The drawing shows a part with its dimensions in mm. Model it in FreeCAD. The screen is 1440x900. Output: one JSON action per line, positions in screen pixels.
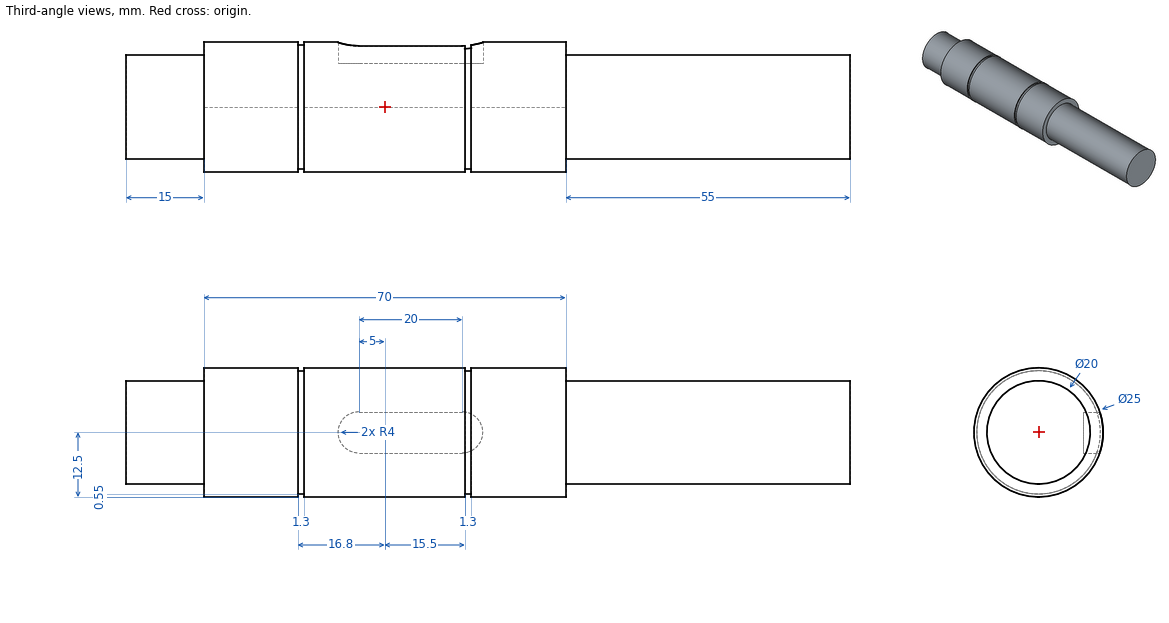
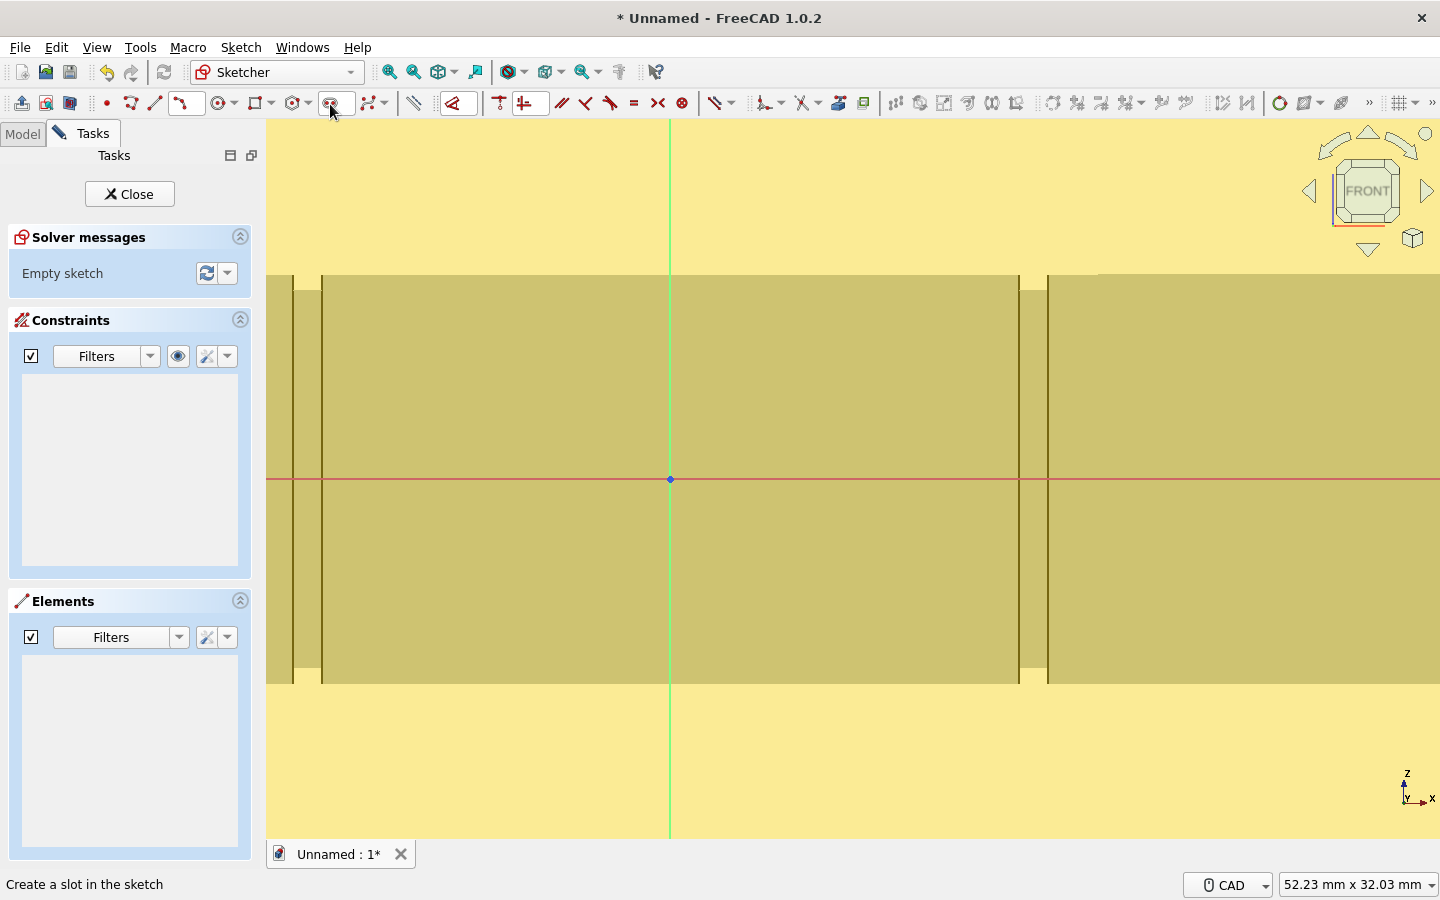
{"action": "left_click", "coordinate": [558, 479]}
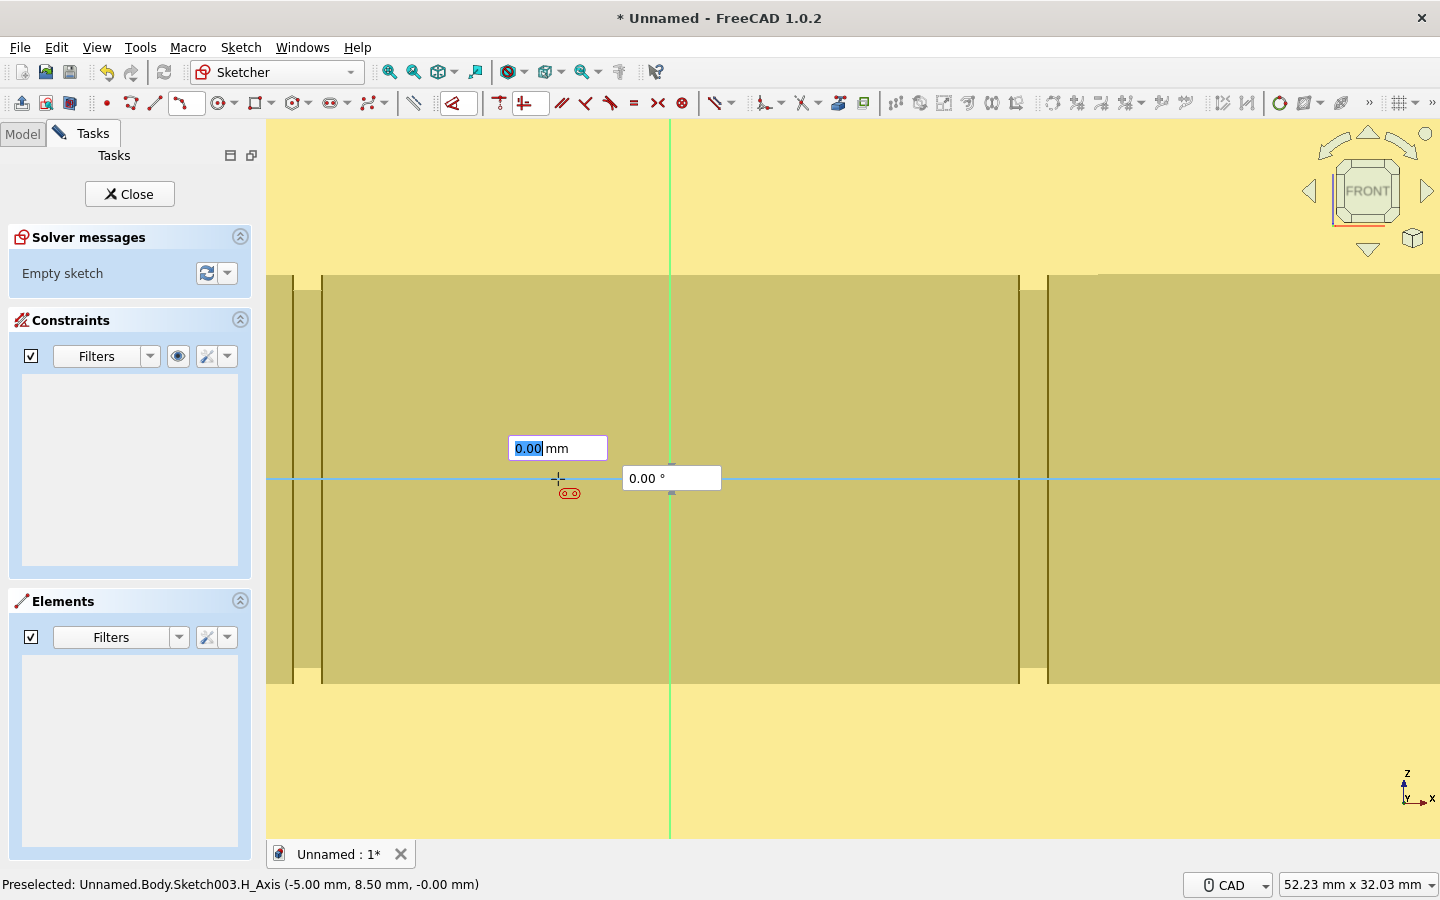
{"action": "left_click", "coordinate": [1007, 470]}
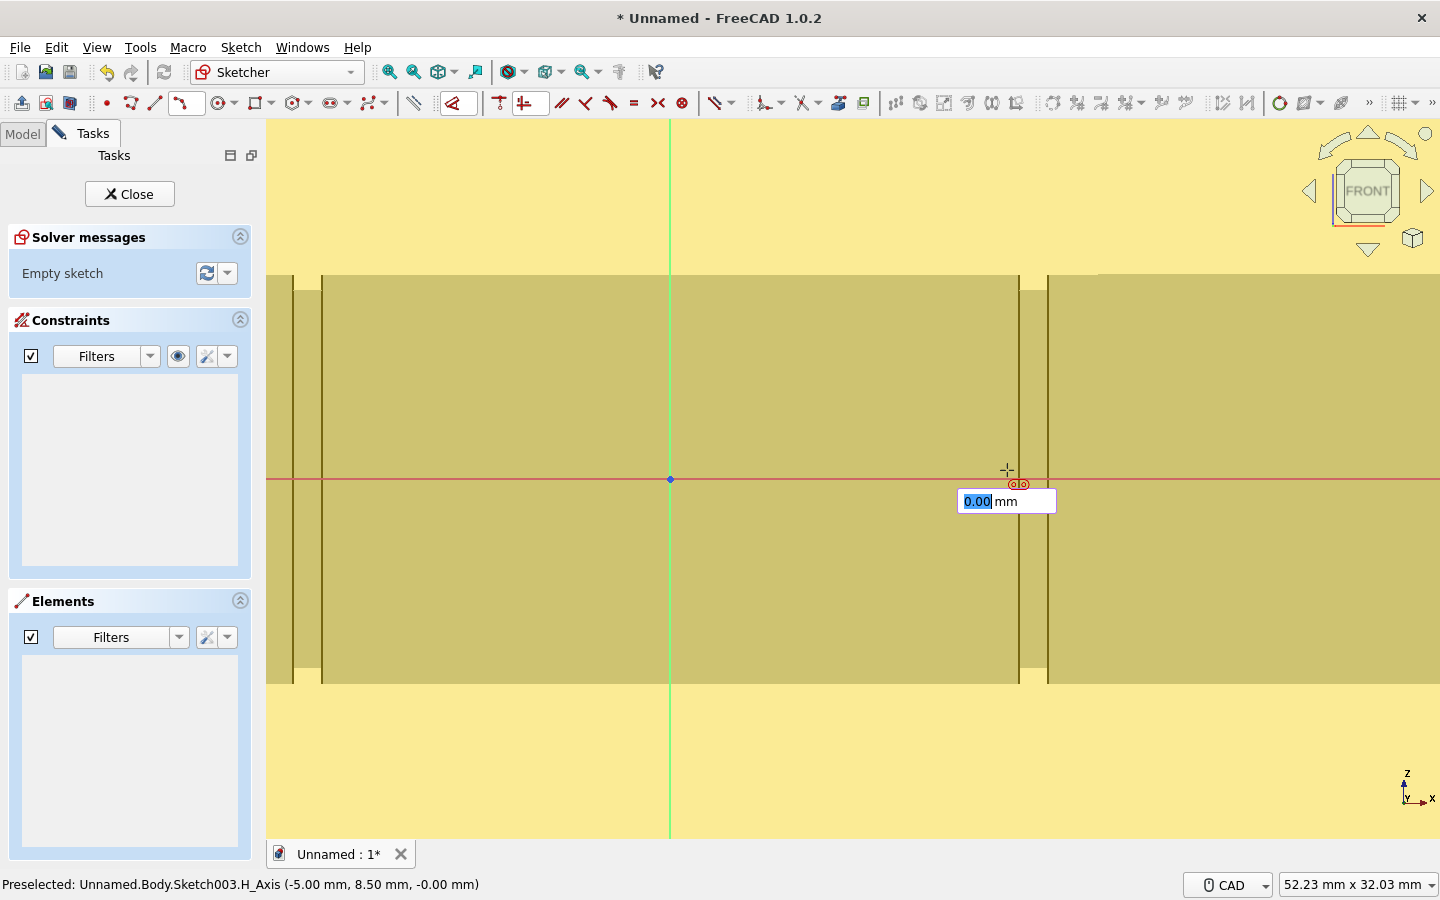
{"action": "left_click", "coordinate": [783, 569]}
{"action": "key", "text": "Escape"}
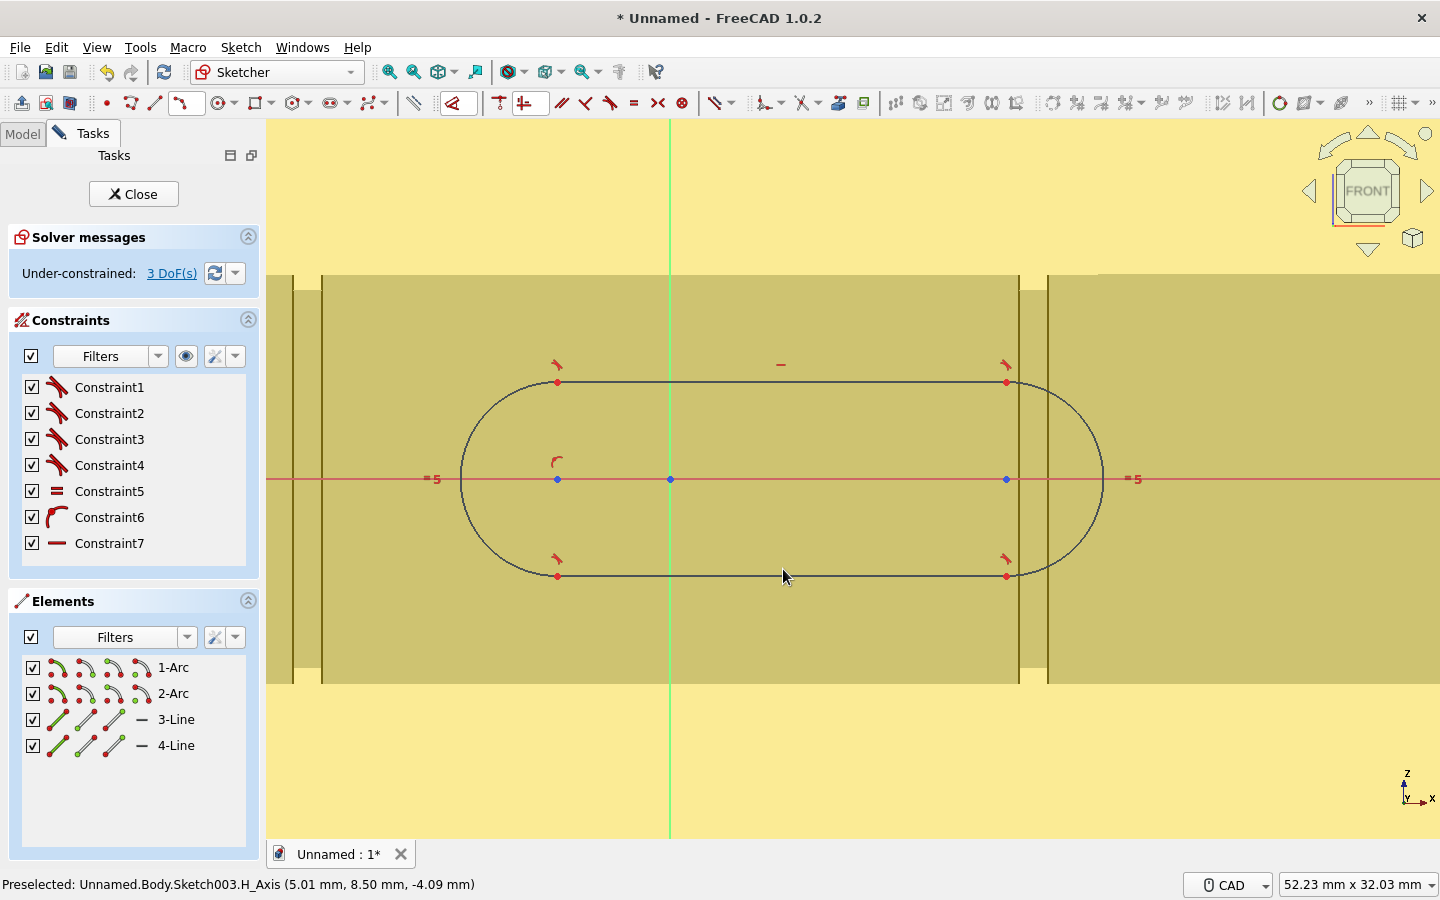
{"action": "left_click", "coordinate": [479, 422]}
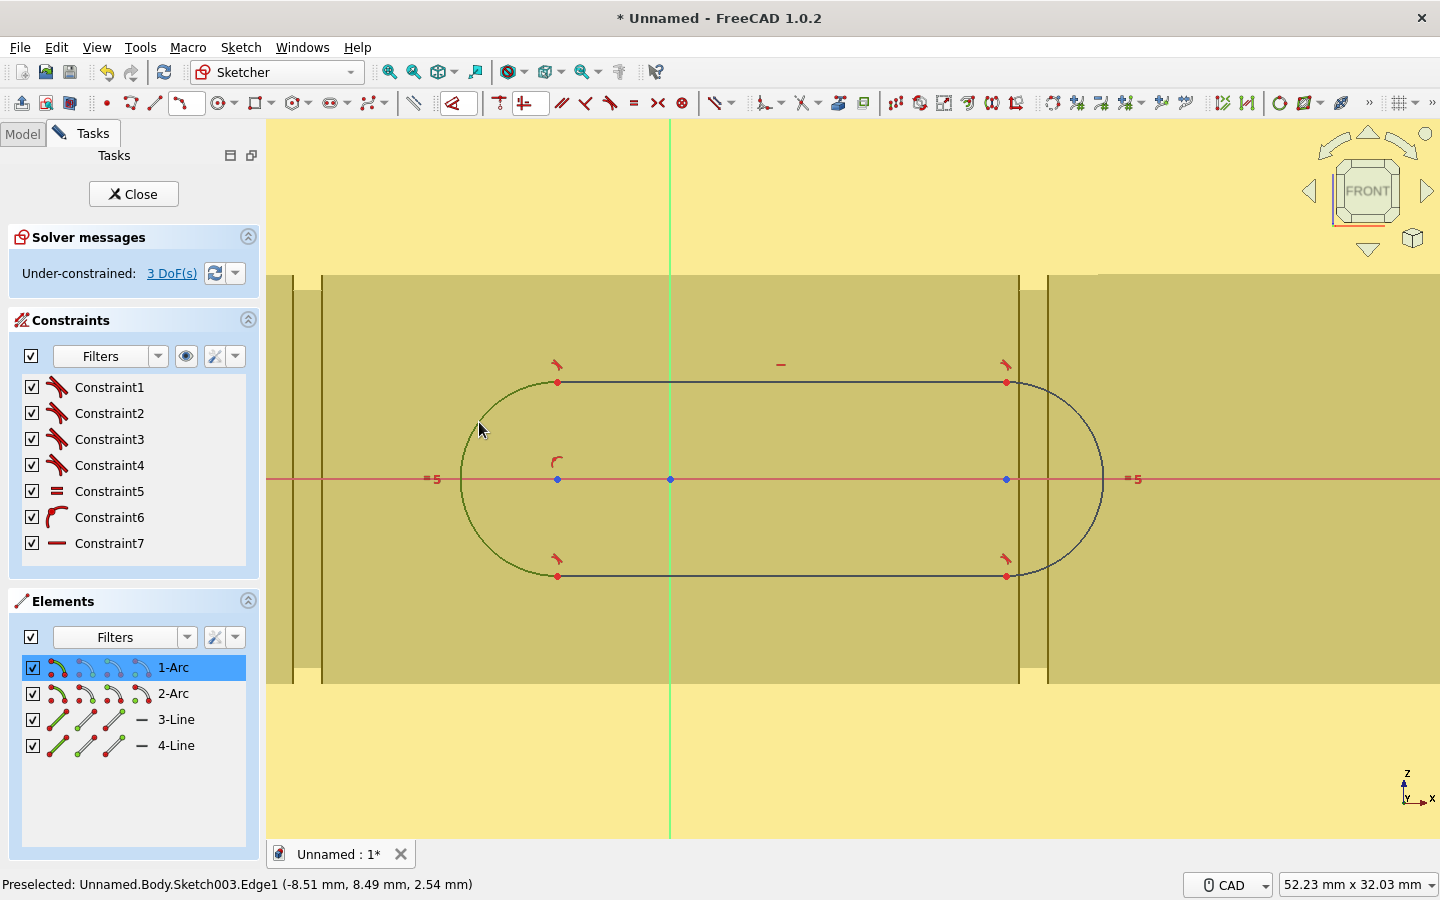
{"action": "left_click", "coordinate": [472, 104]}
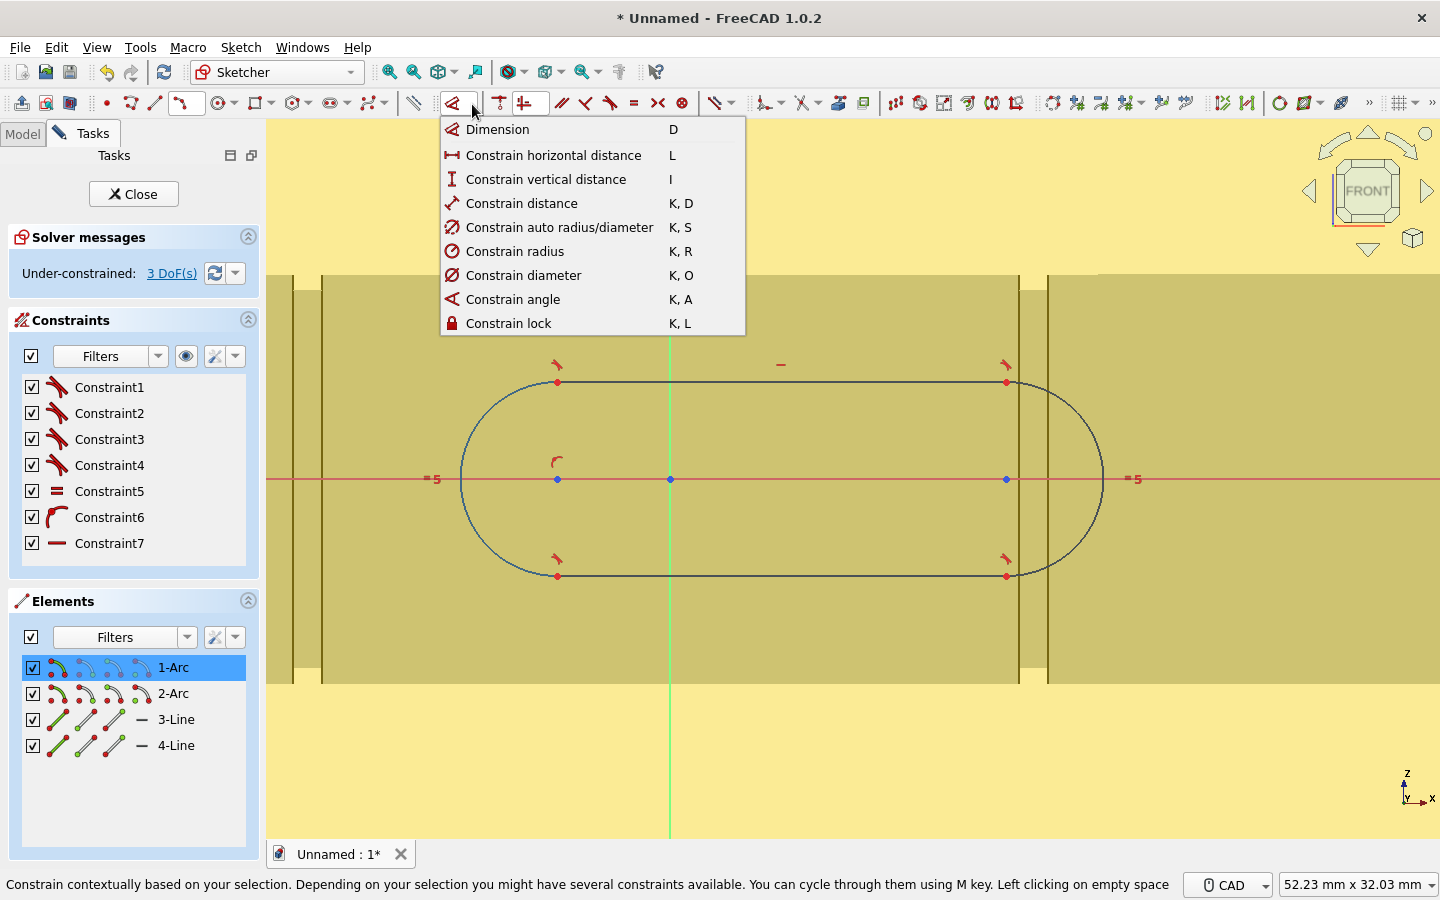
{"action": "left_click", "coordinate": [593, 251]}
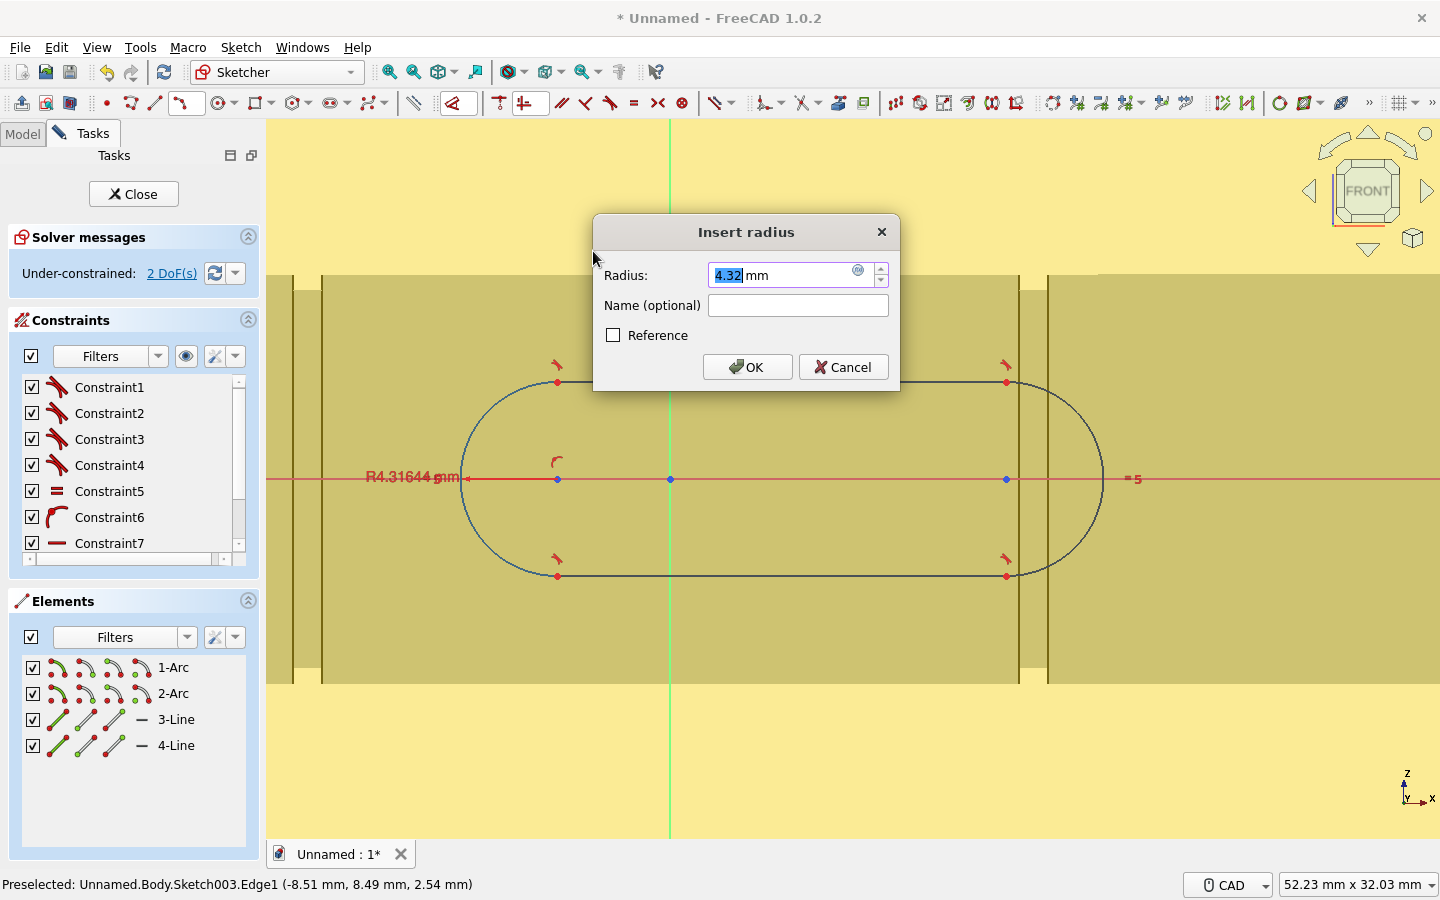
{"action": "type", "text": "4"}
{"action": "key", "text": "Return"}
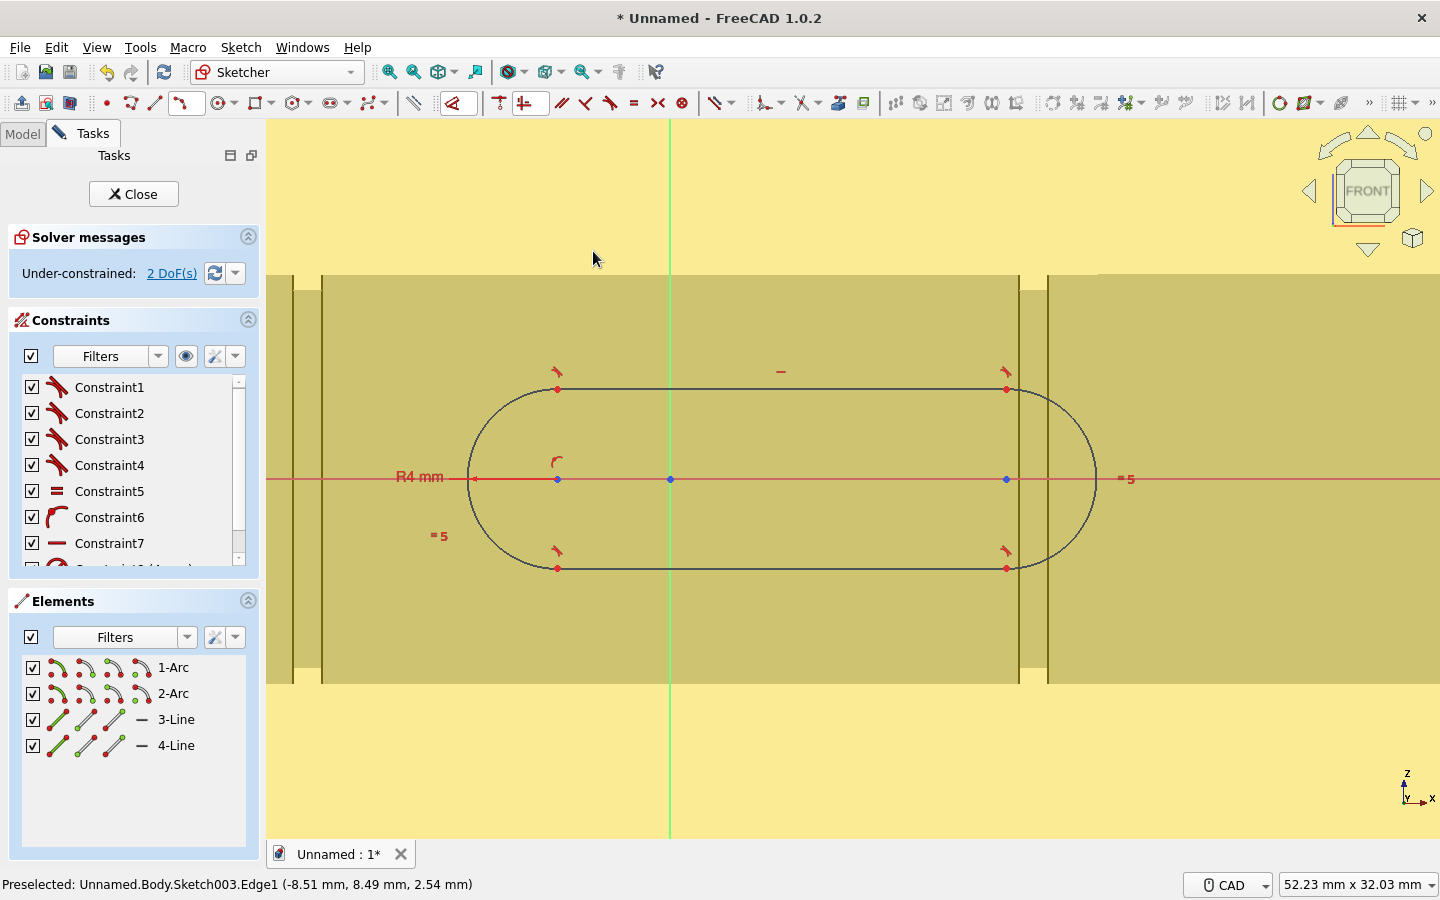
{"action": "left_click", "coordinate": [692, 389]}